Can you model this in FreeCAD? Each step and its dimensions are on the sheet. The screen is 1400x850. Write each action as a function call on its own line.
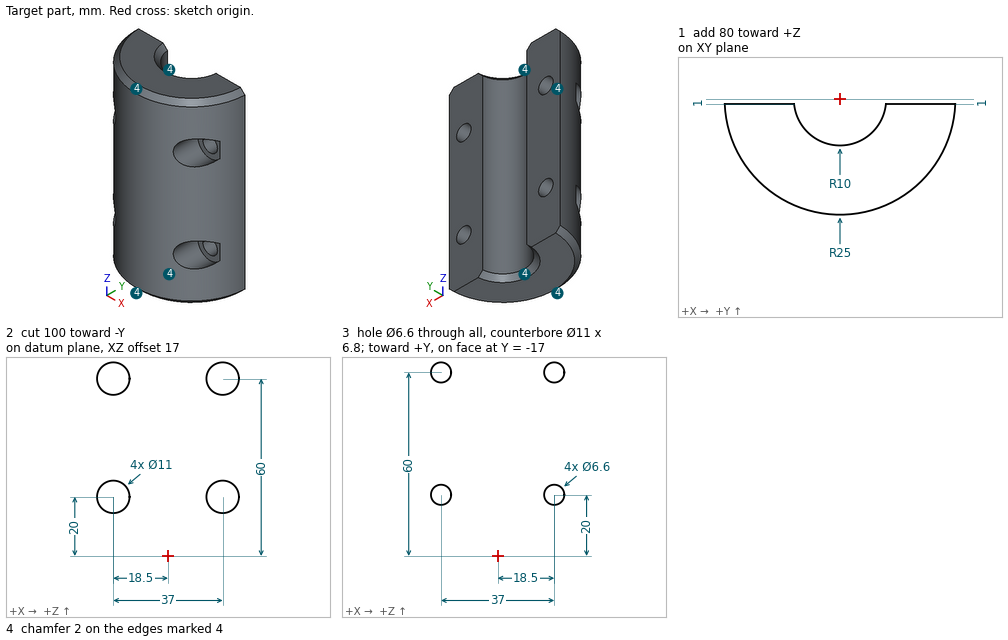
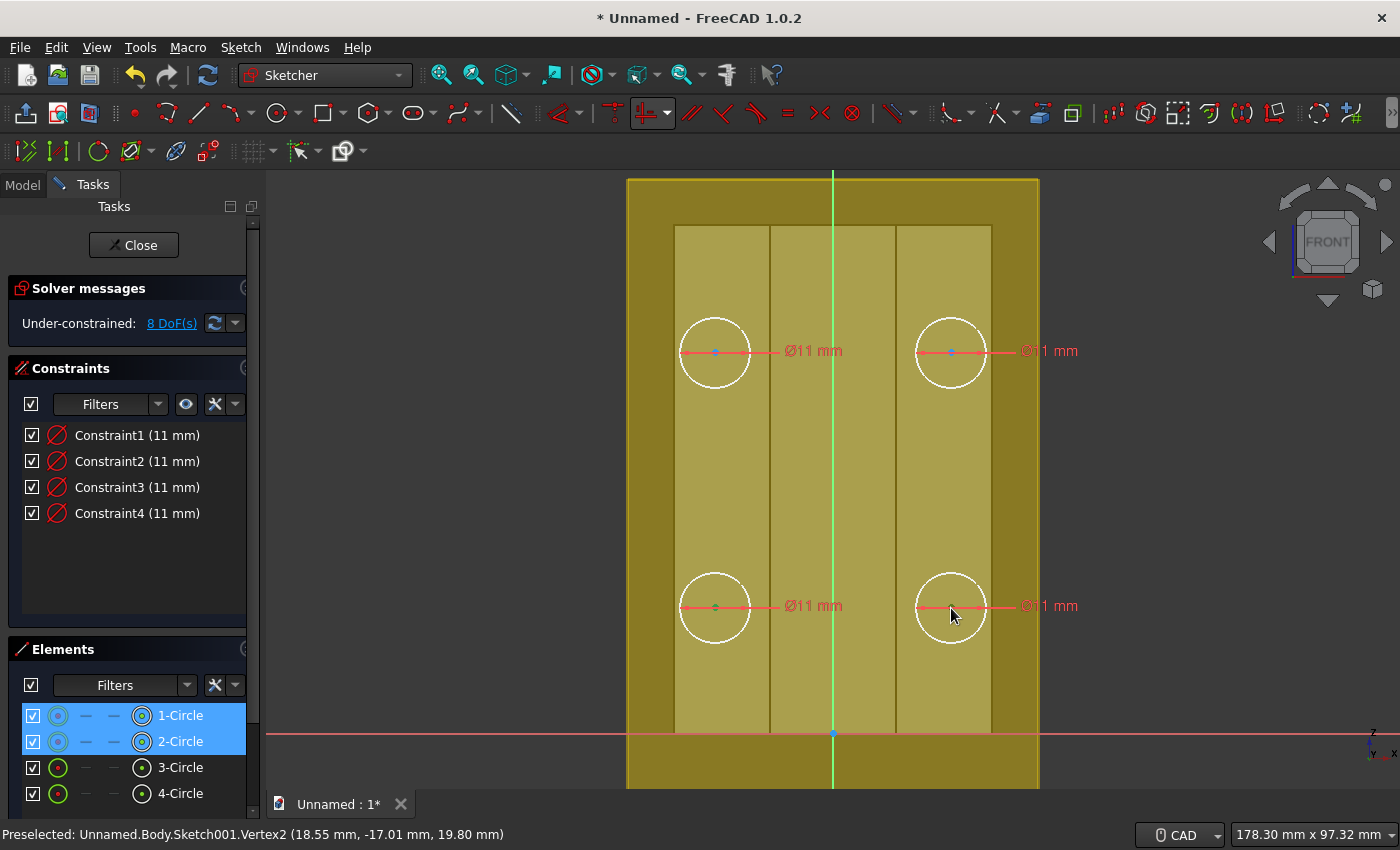
key(h)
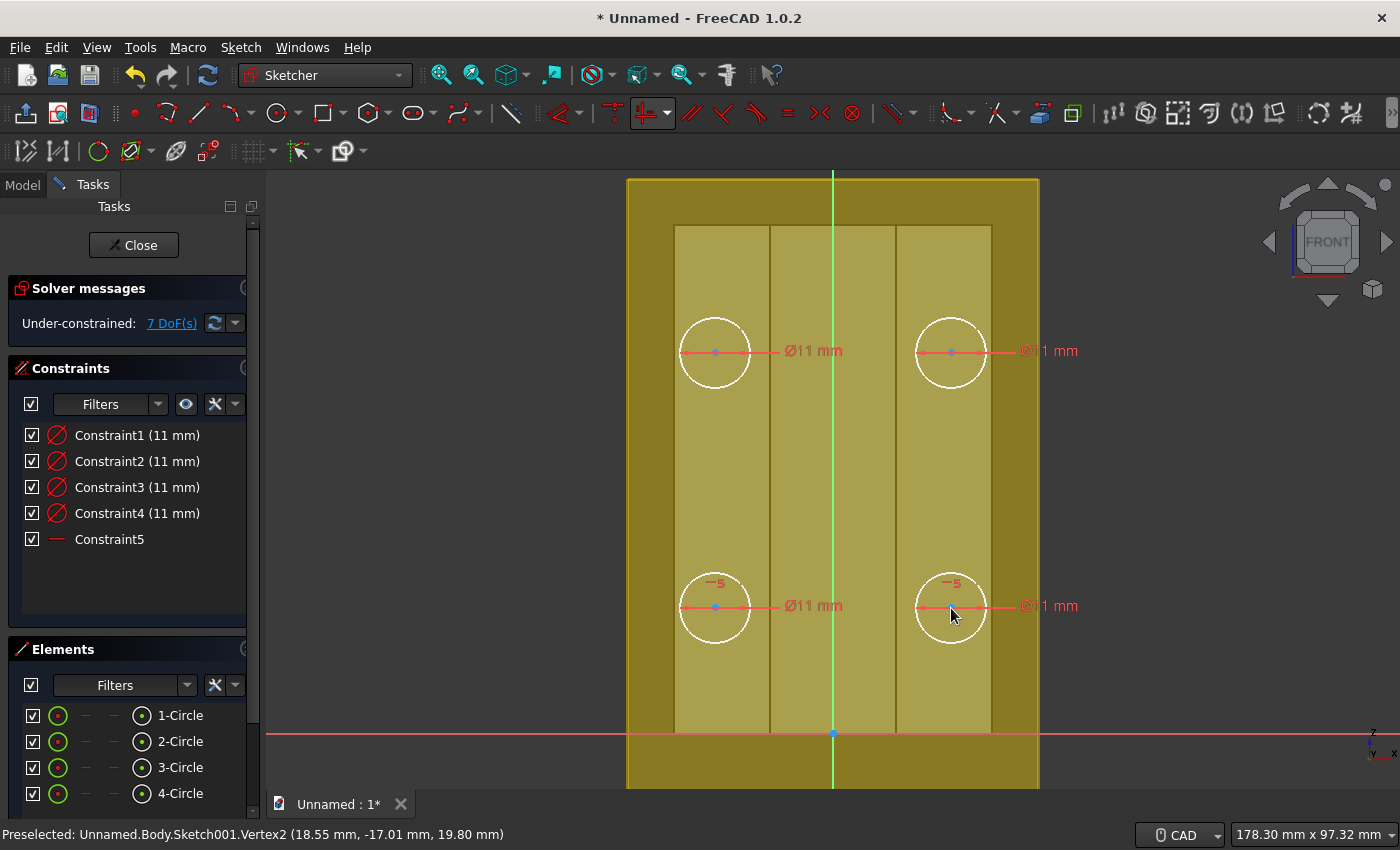
click(951, 608)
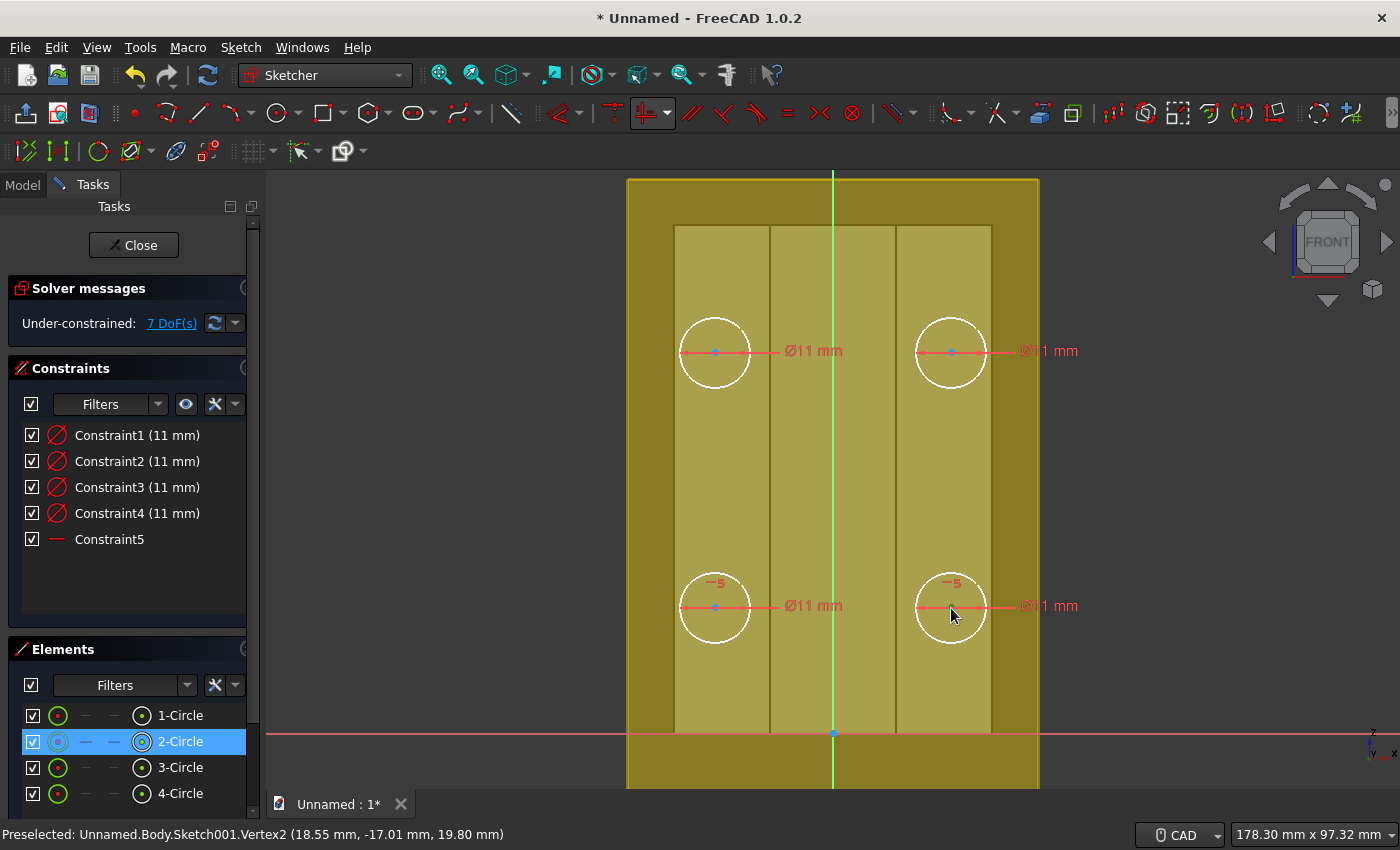
click(951, 353)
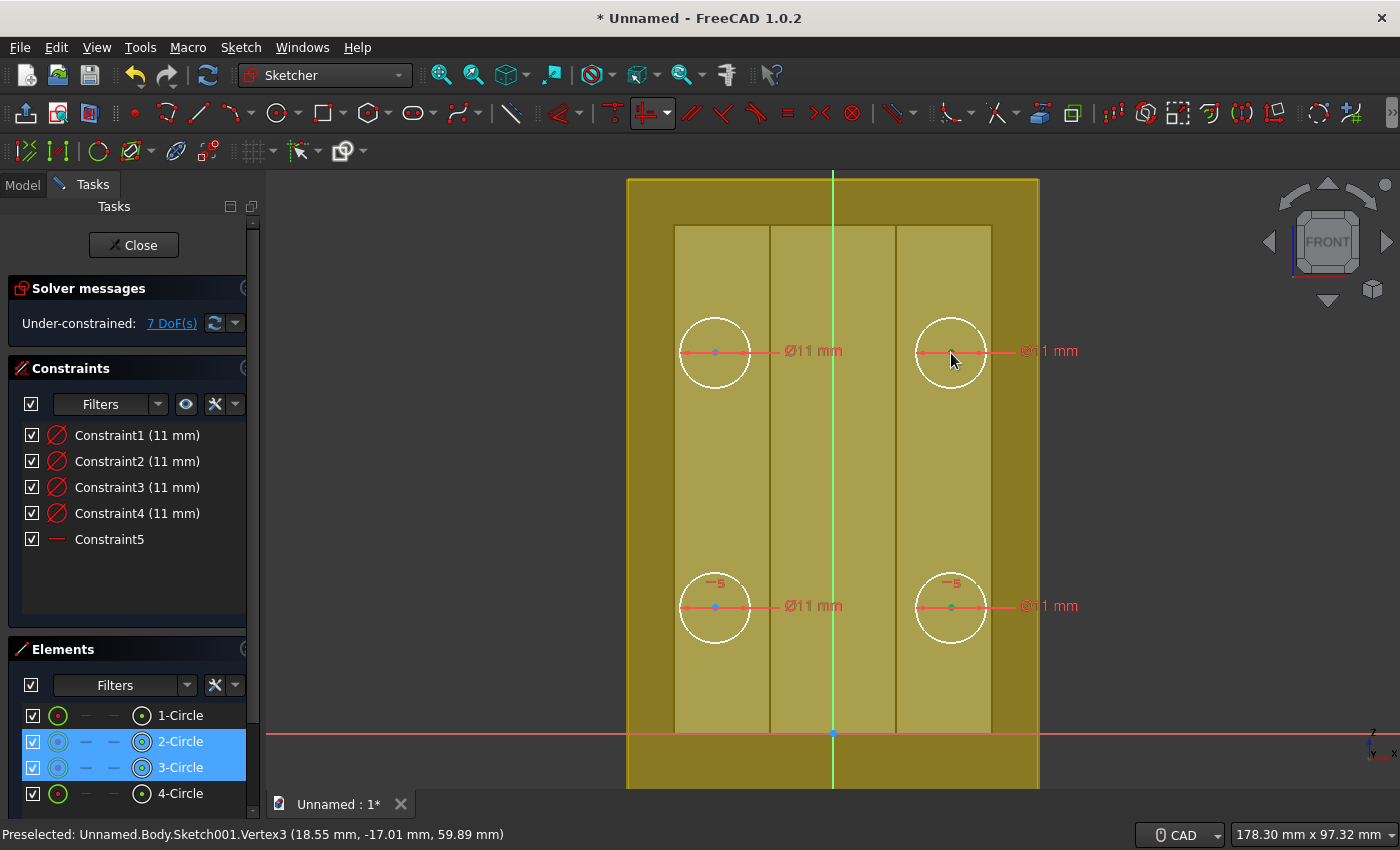
click(670, 114)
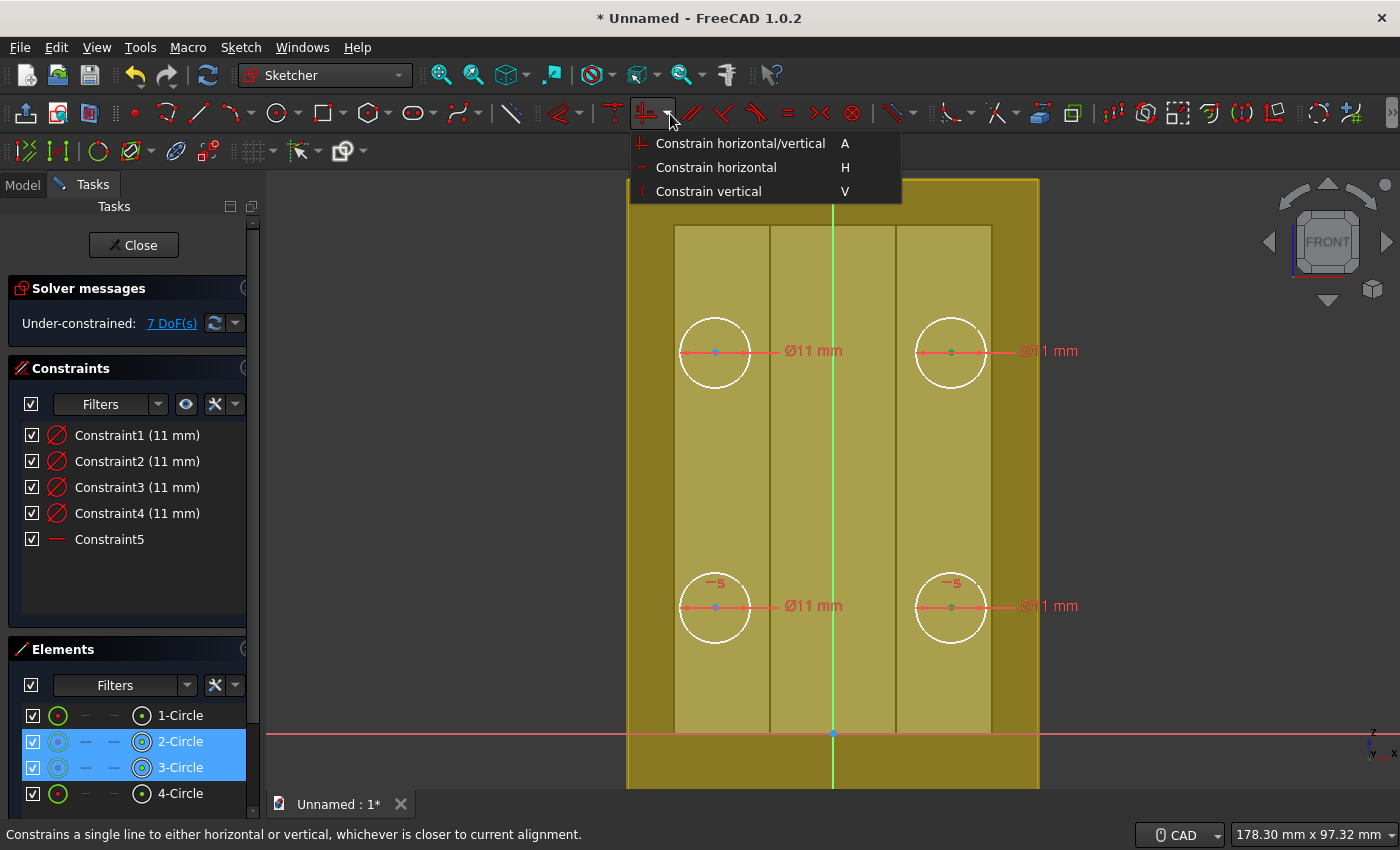
click(766, 191)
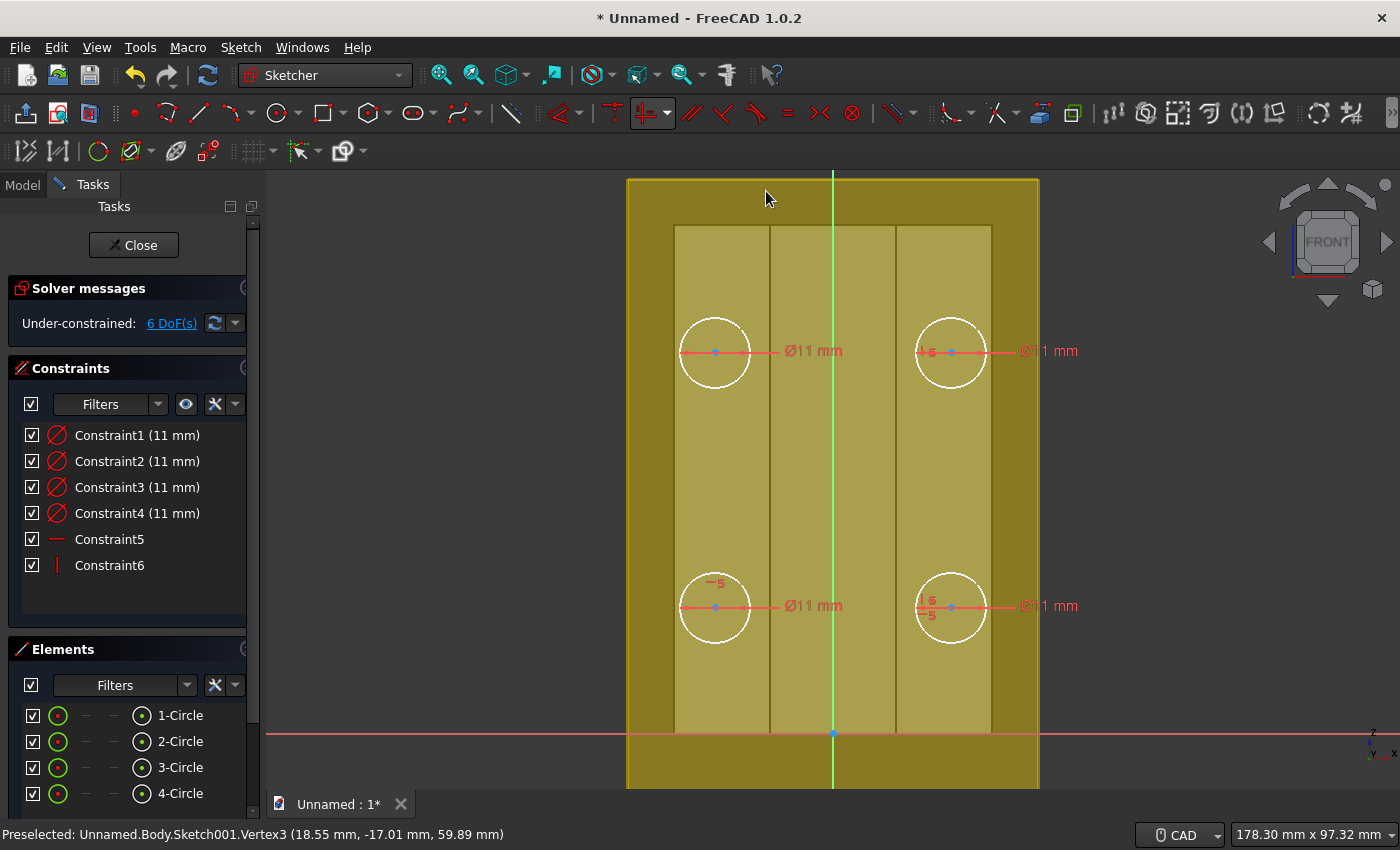
click(715, 608)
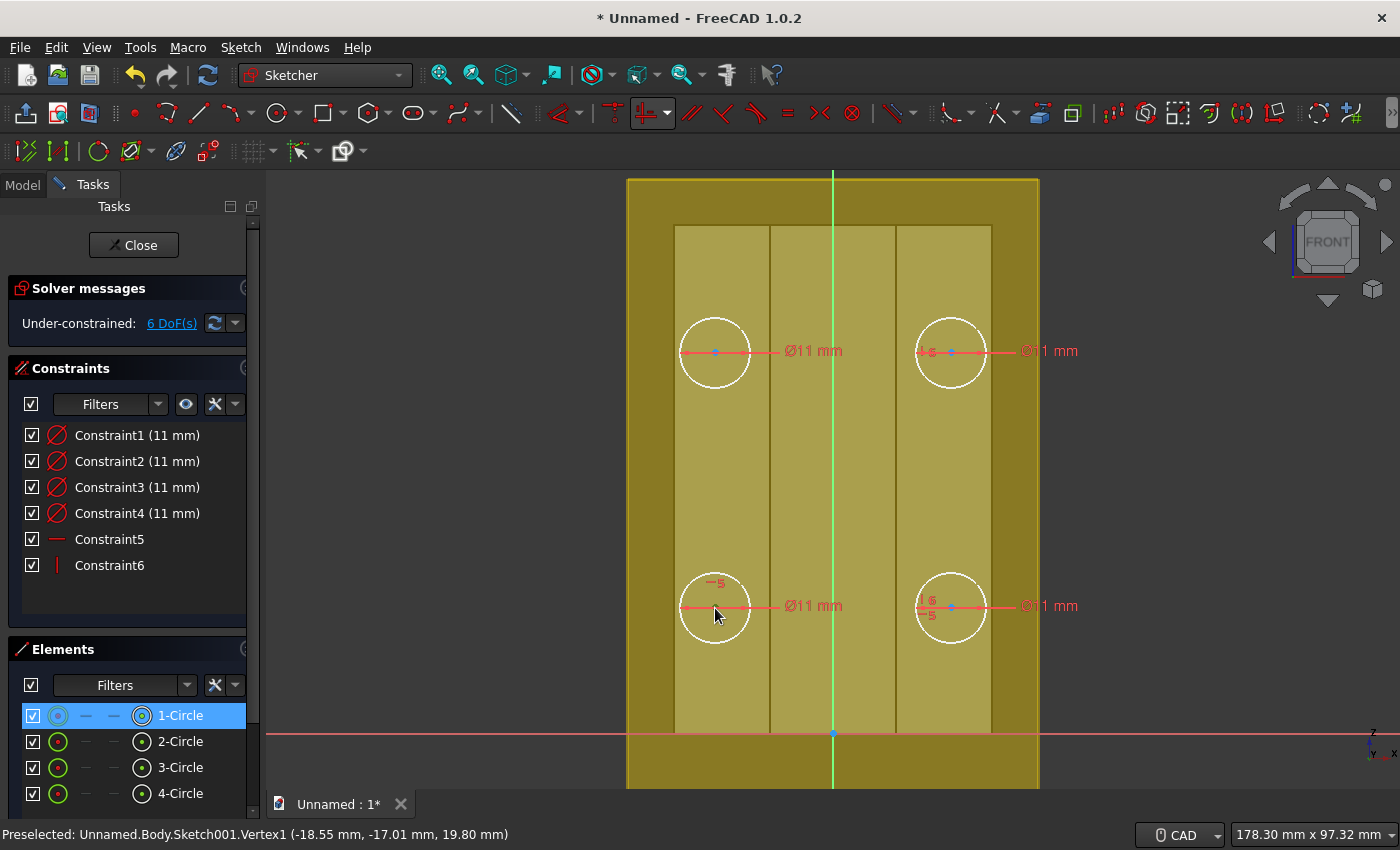
click(715, 353)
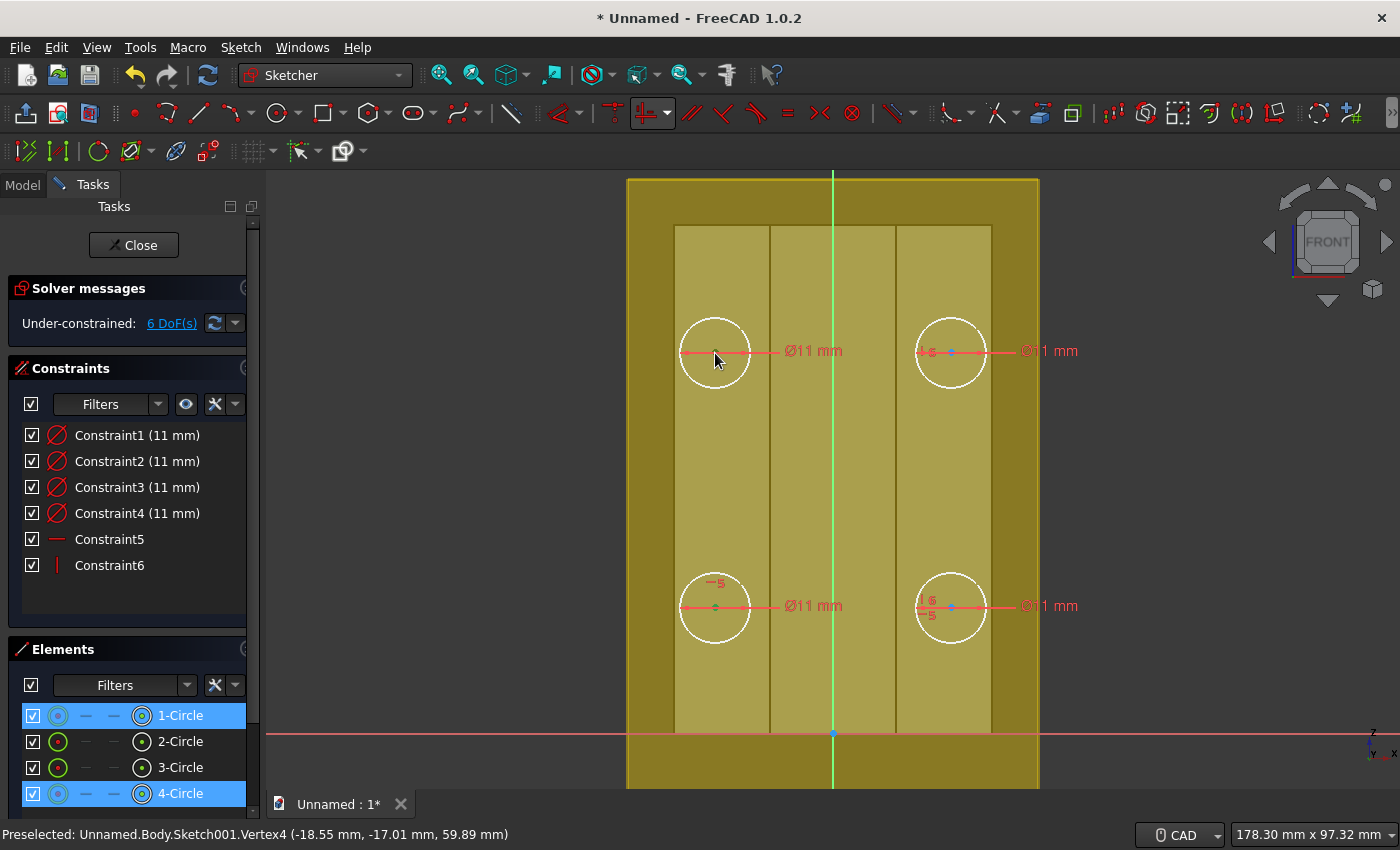
click(670, 114)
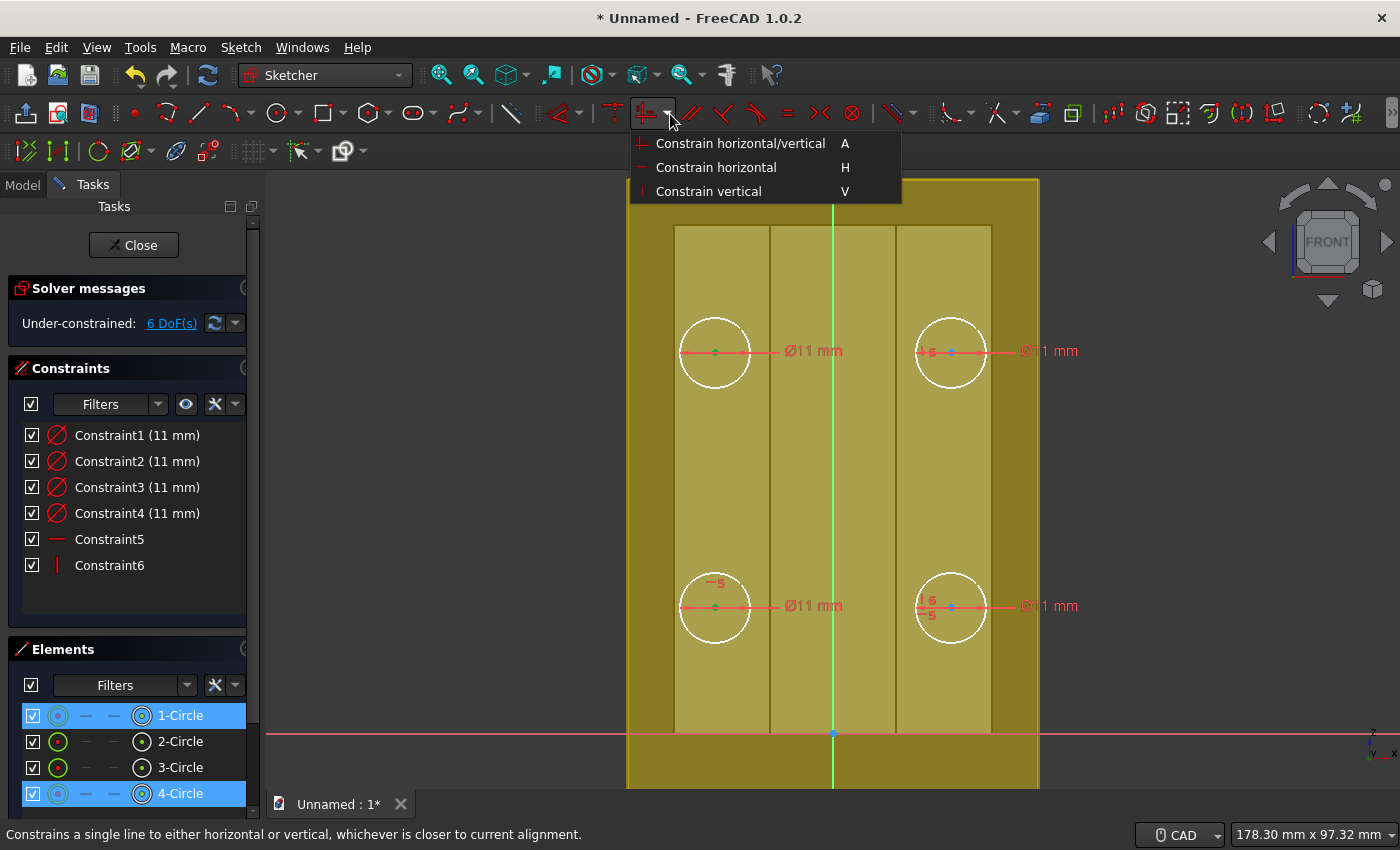
click(766, 191)